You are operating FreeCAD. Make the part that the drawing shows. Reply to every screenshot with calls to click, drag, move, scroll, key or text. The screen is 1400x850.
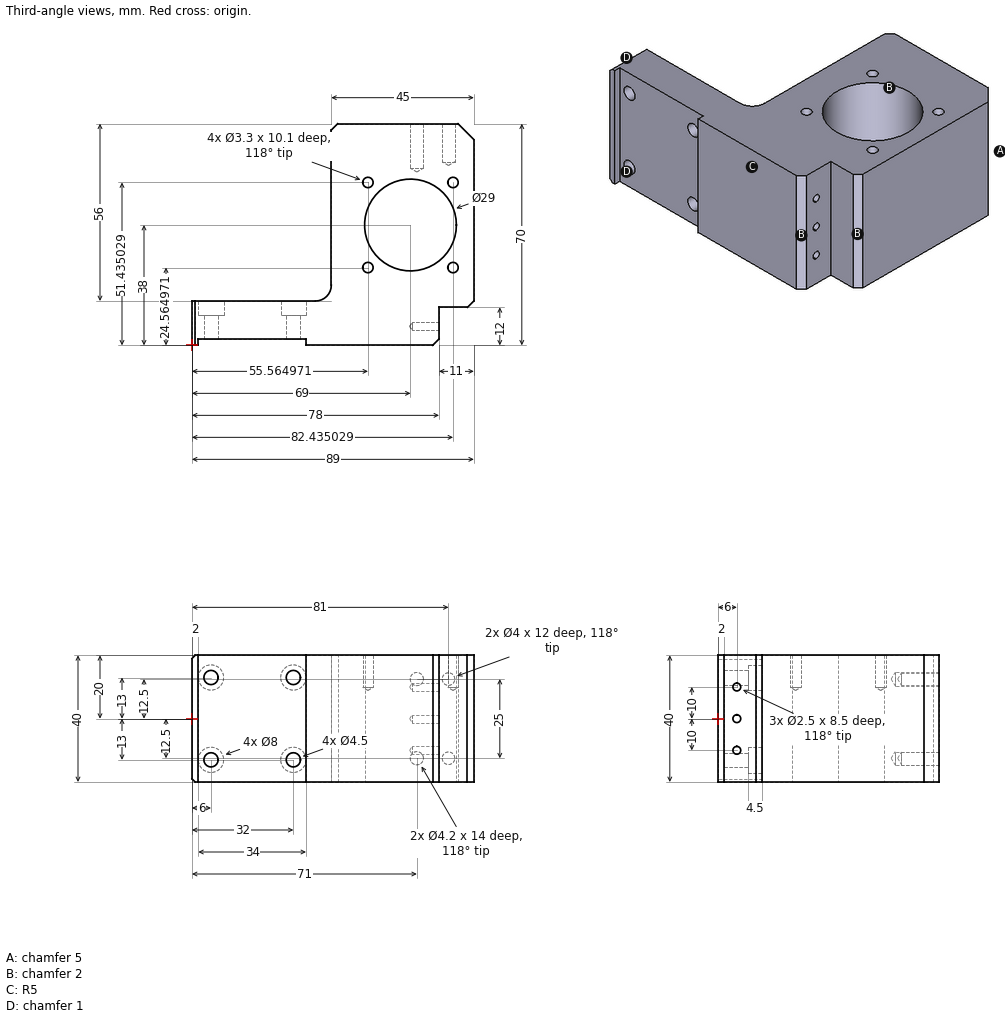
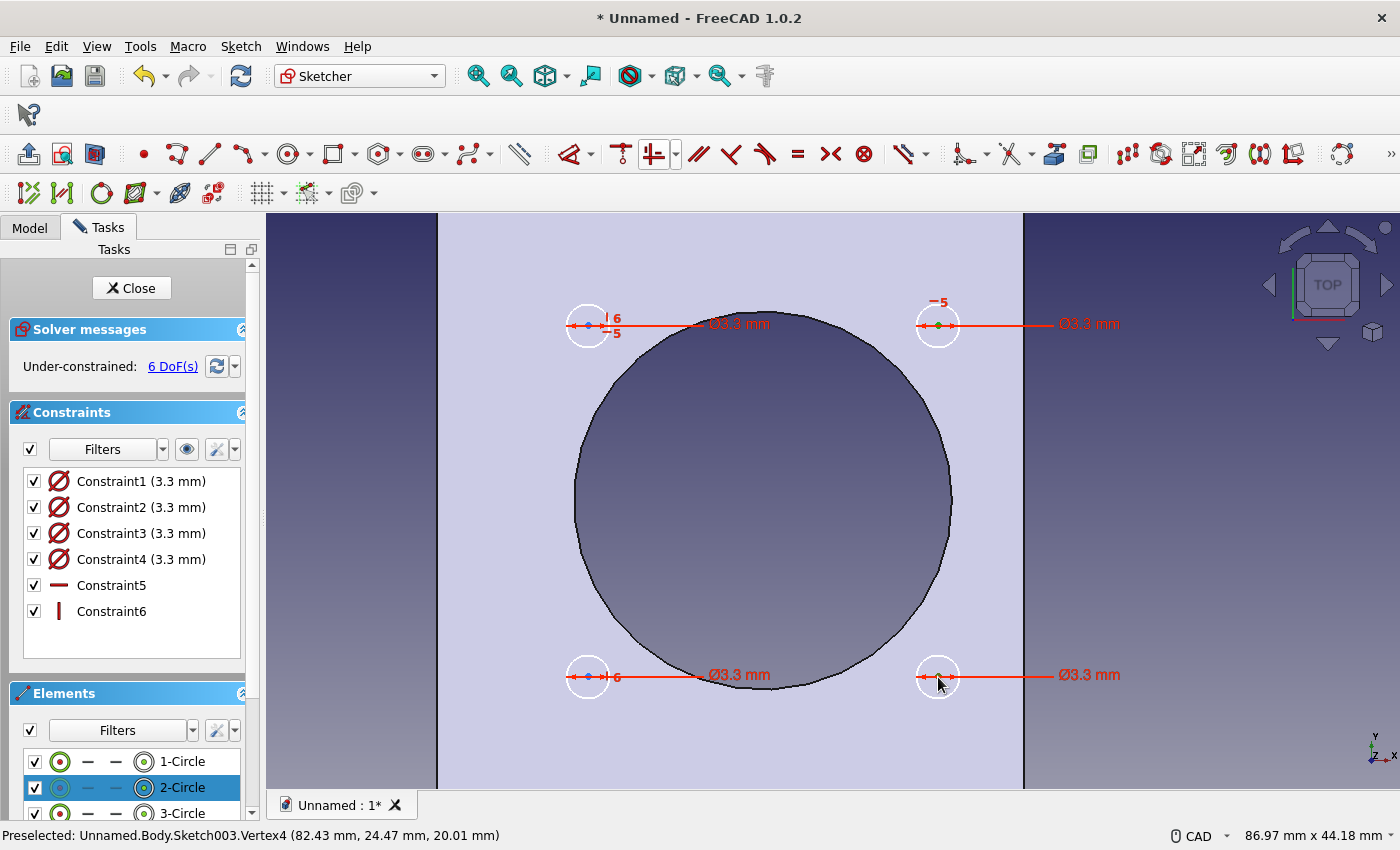
key(v)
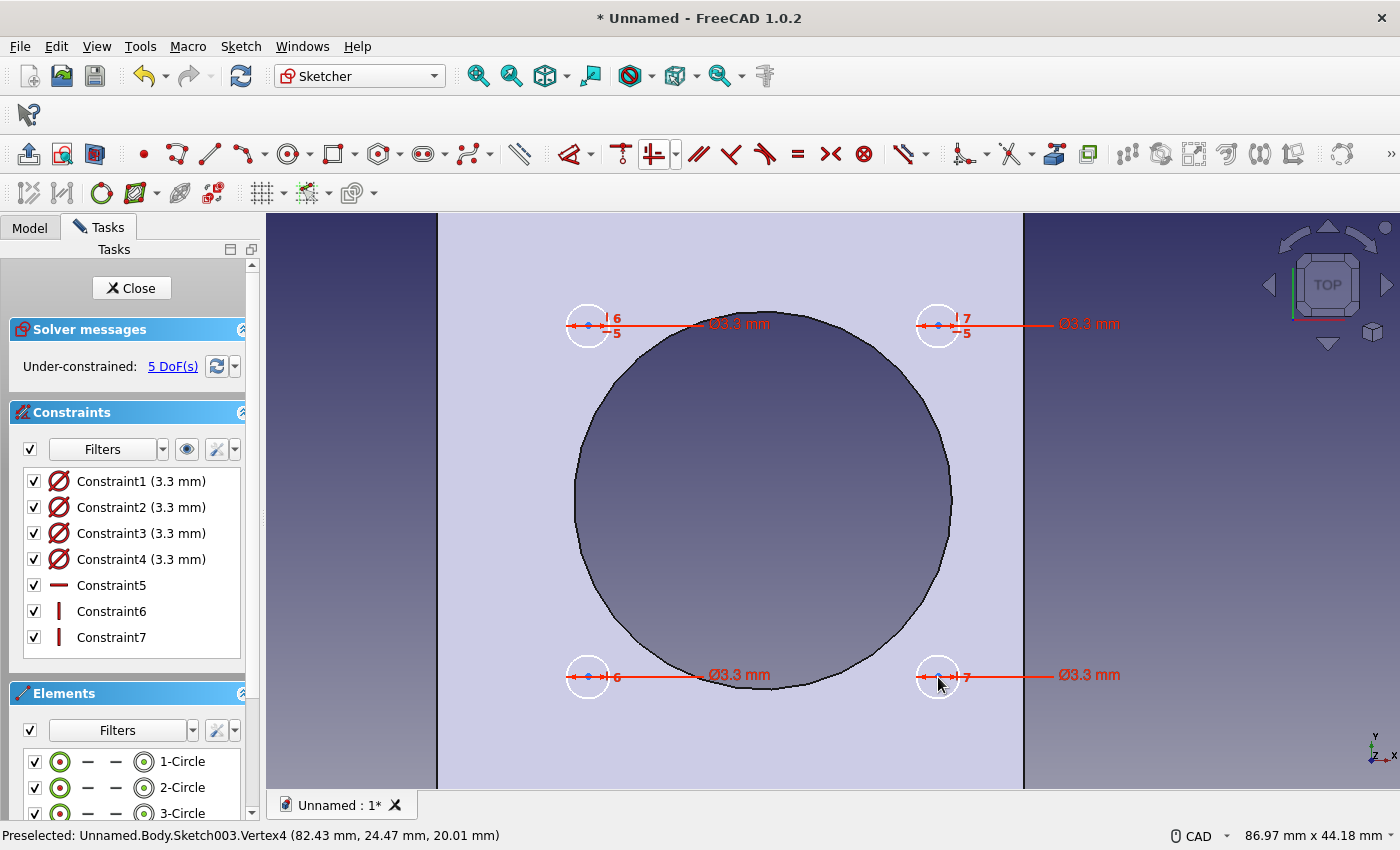
click(588, 677)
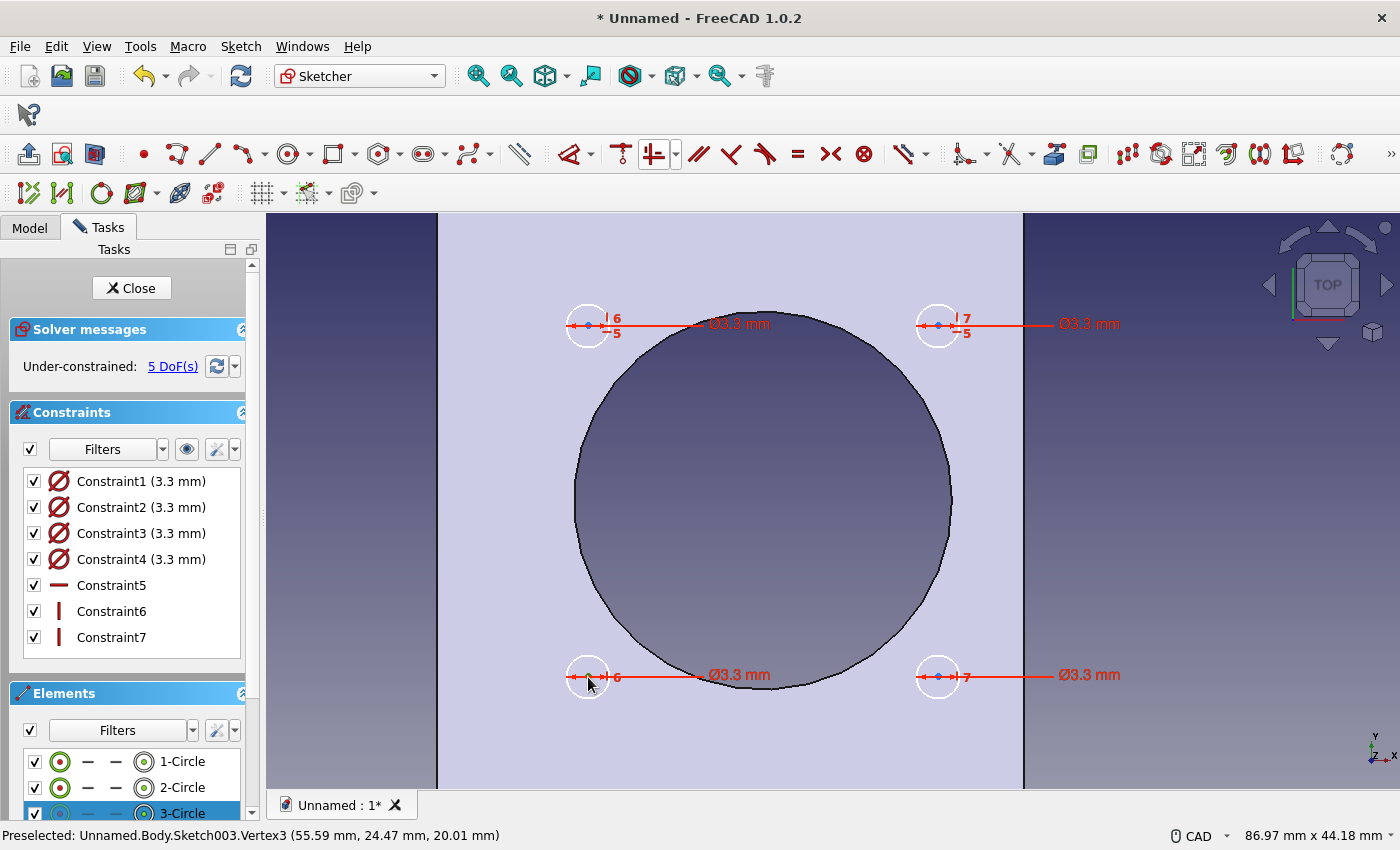
click(938, 677)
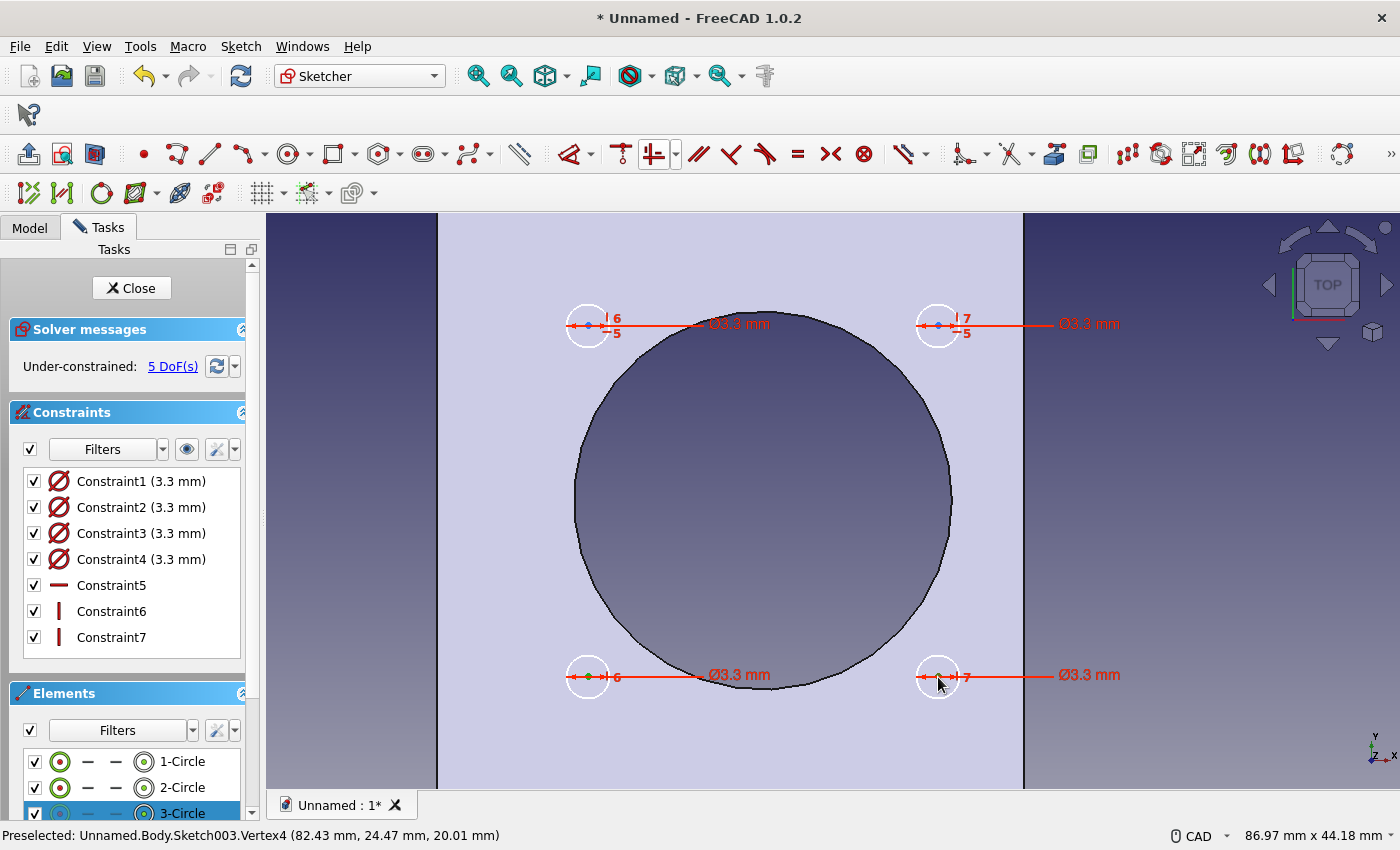
key(h)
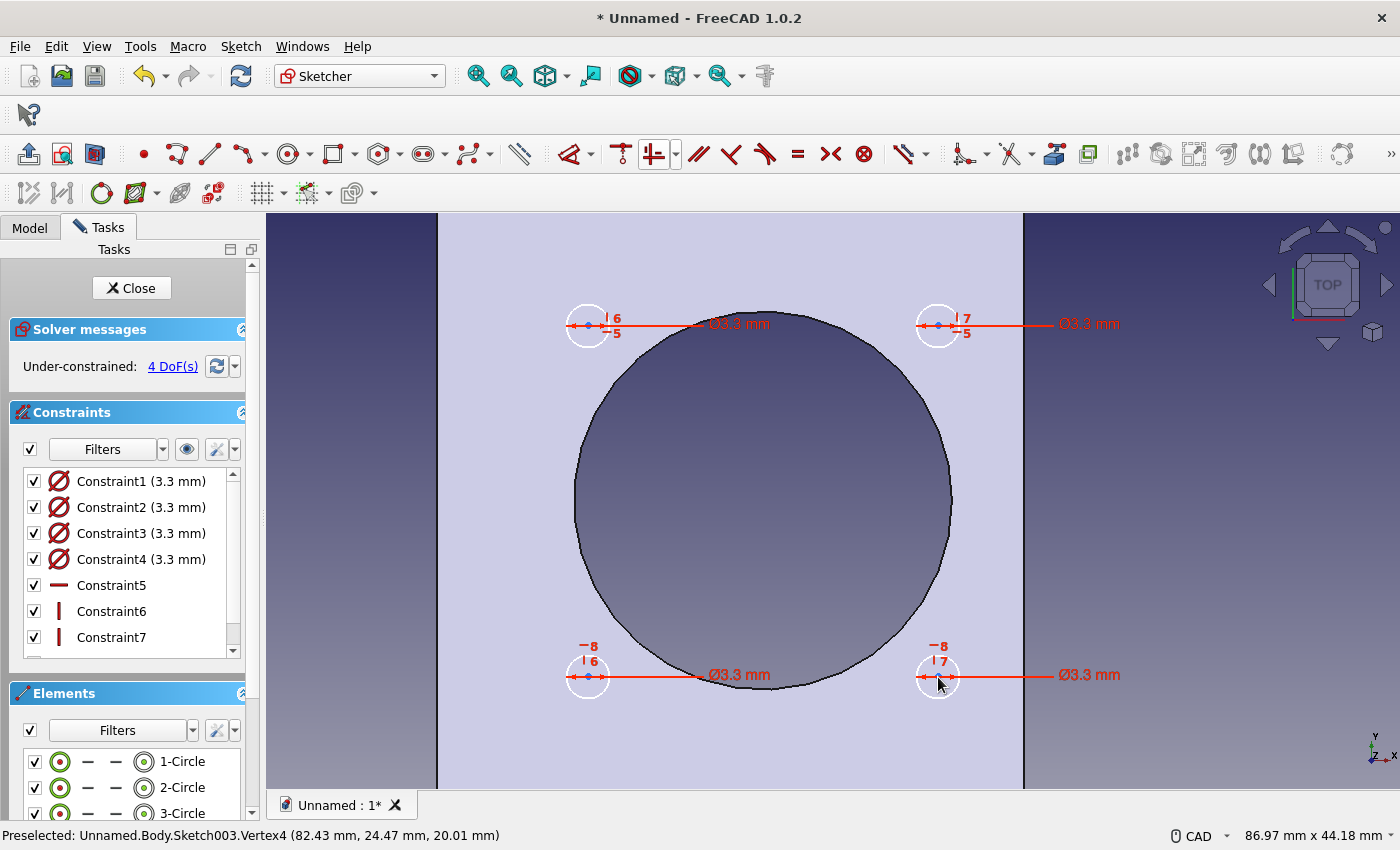
key(d)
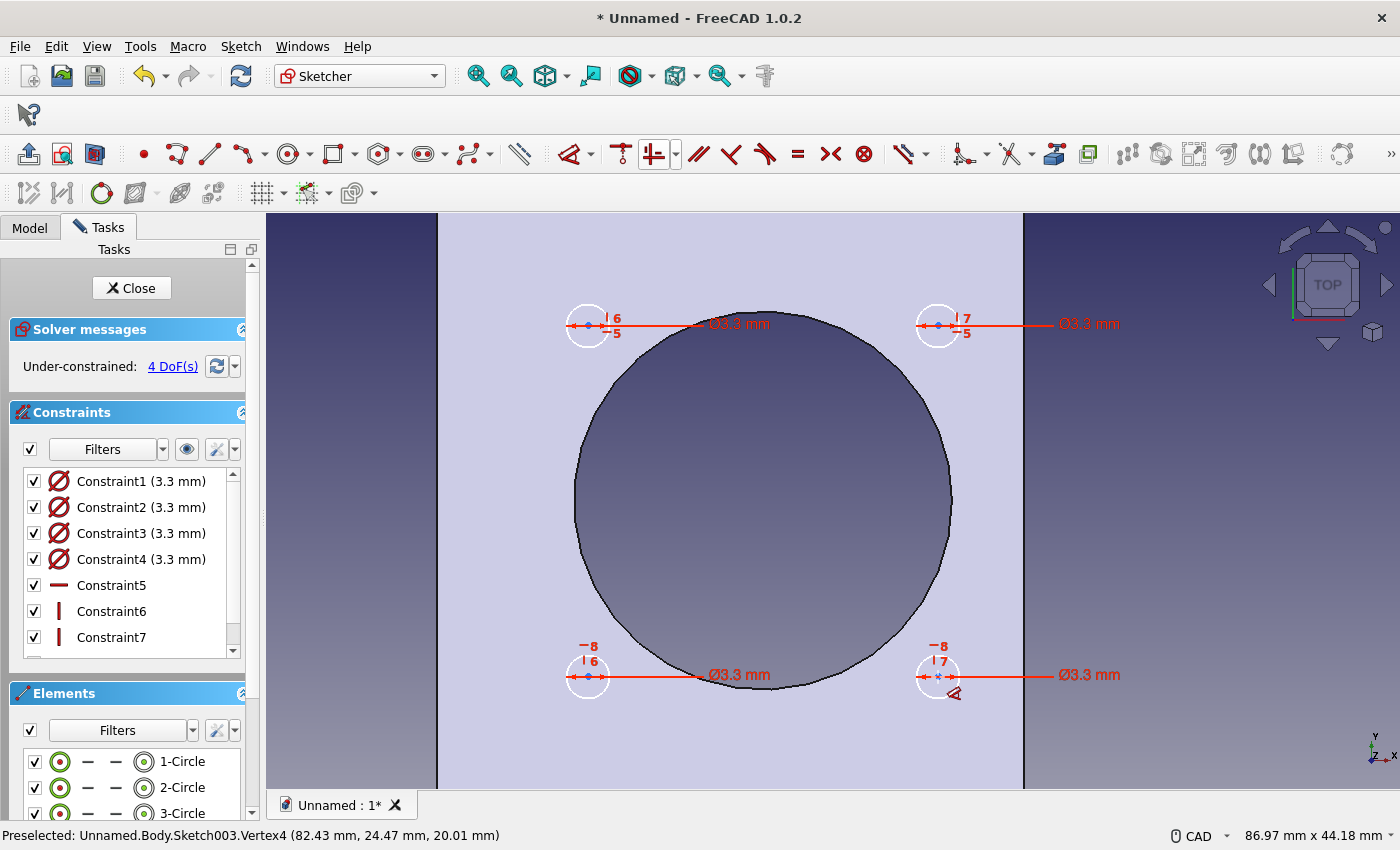
click(588, 326)
click(441, 292)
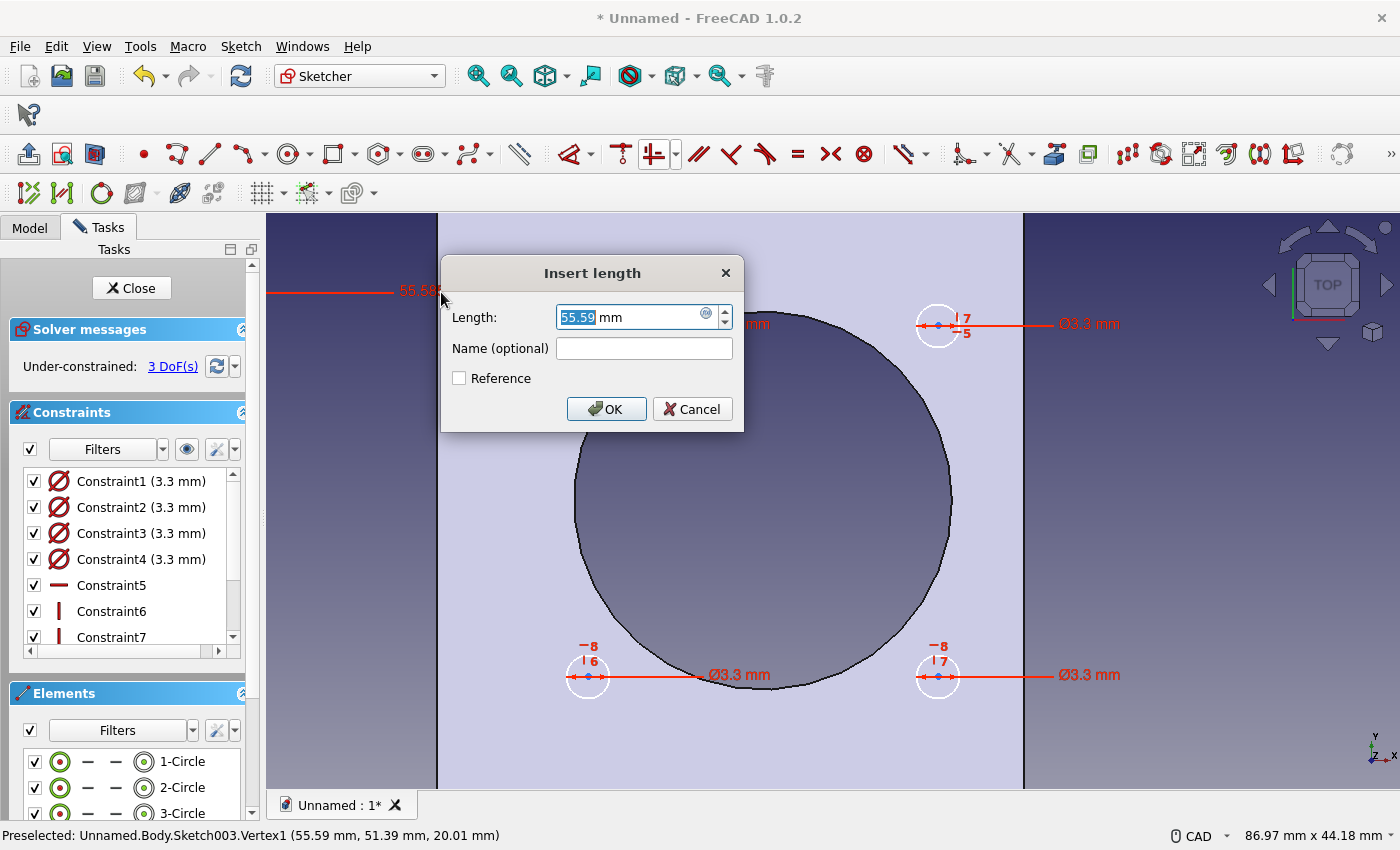
text(55.564971)
key(Return)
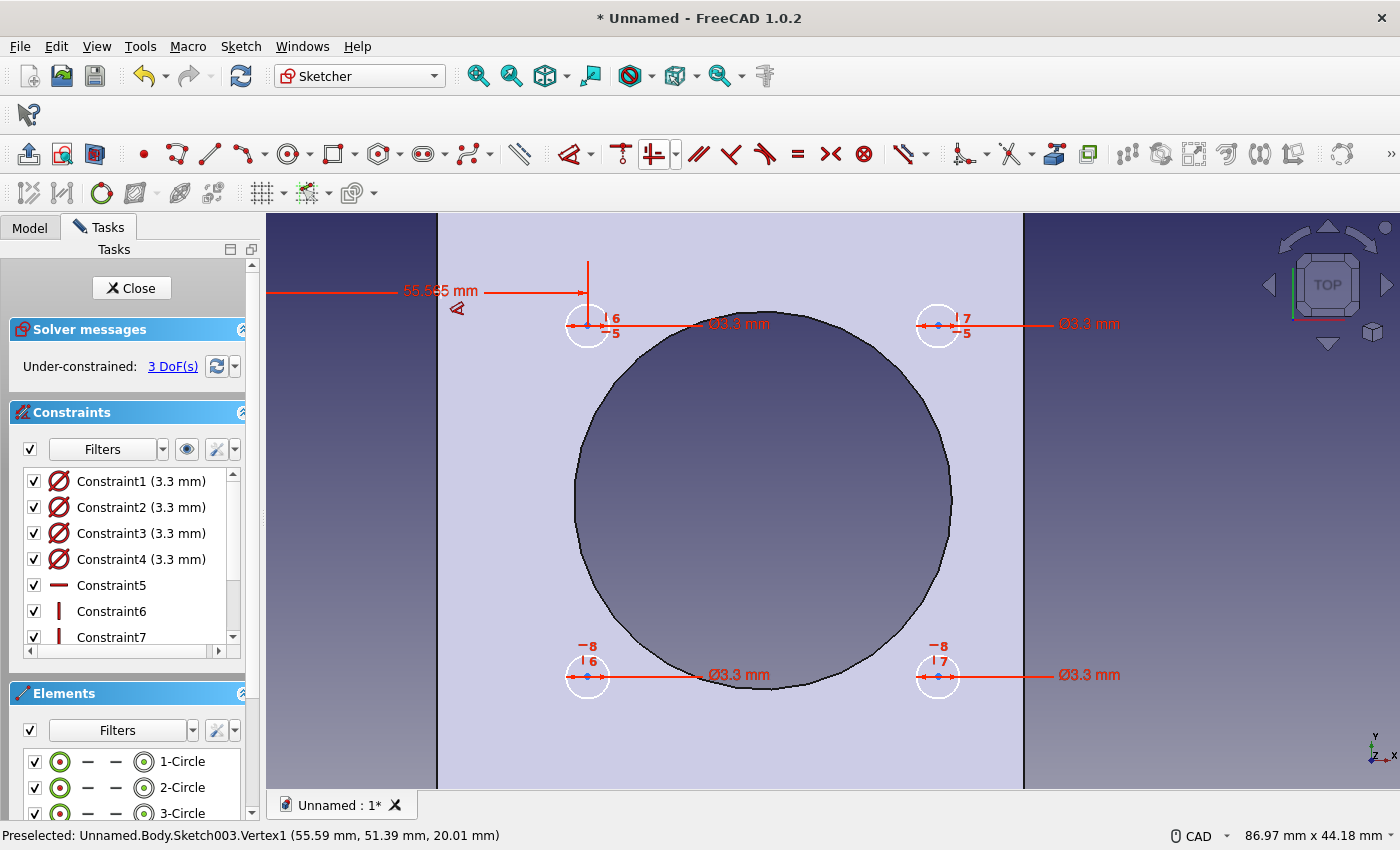
click(588, 326)
click(622, 544)